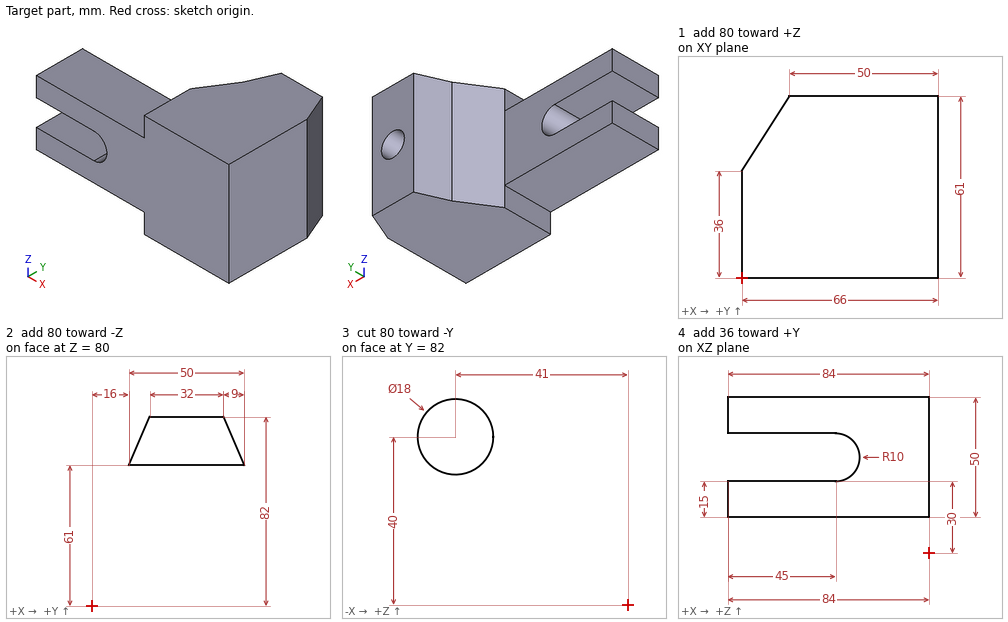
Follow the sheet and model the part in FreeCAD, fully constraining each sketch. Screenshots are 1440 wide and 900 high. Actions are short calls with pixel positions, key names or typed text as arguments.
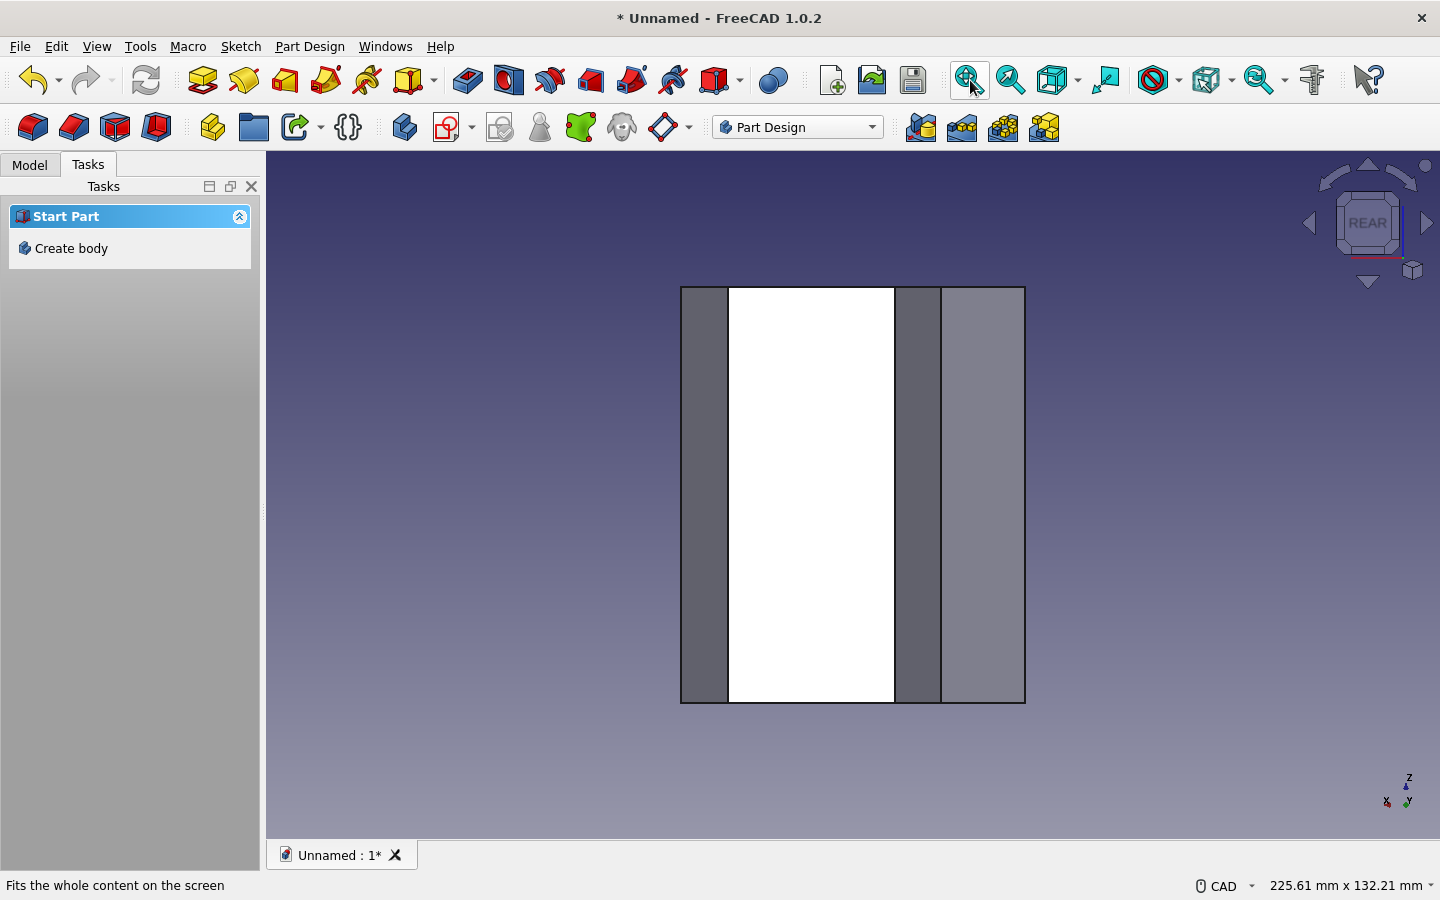
click(811, 375)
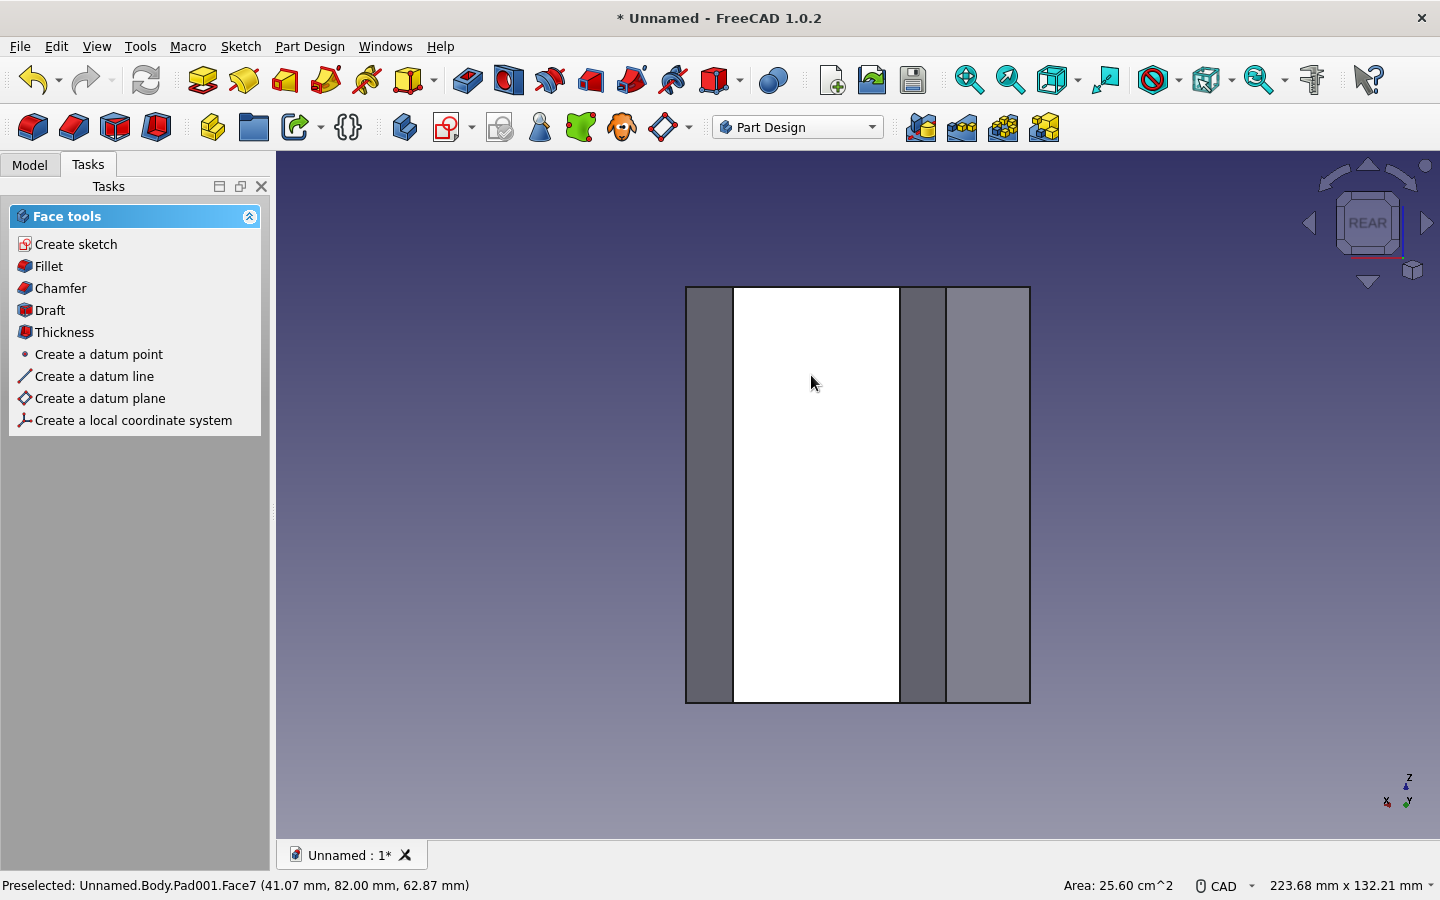
click(446, 128)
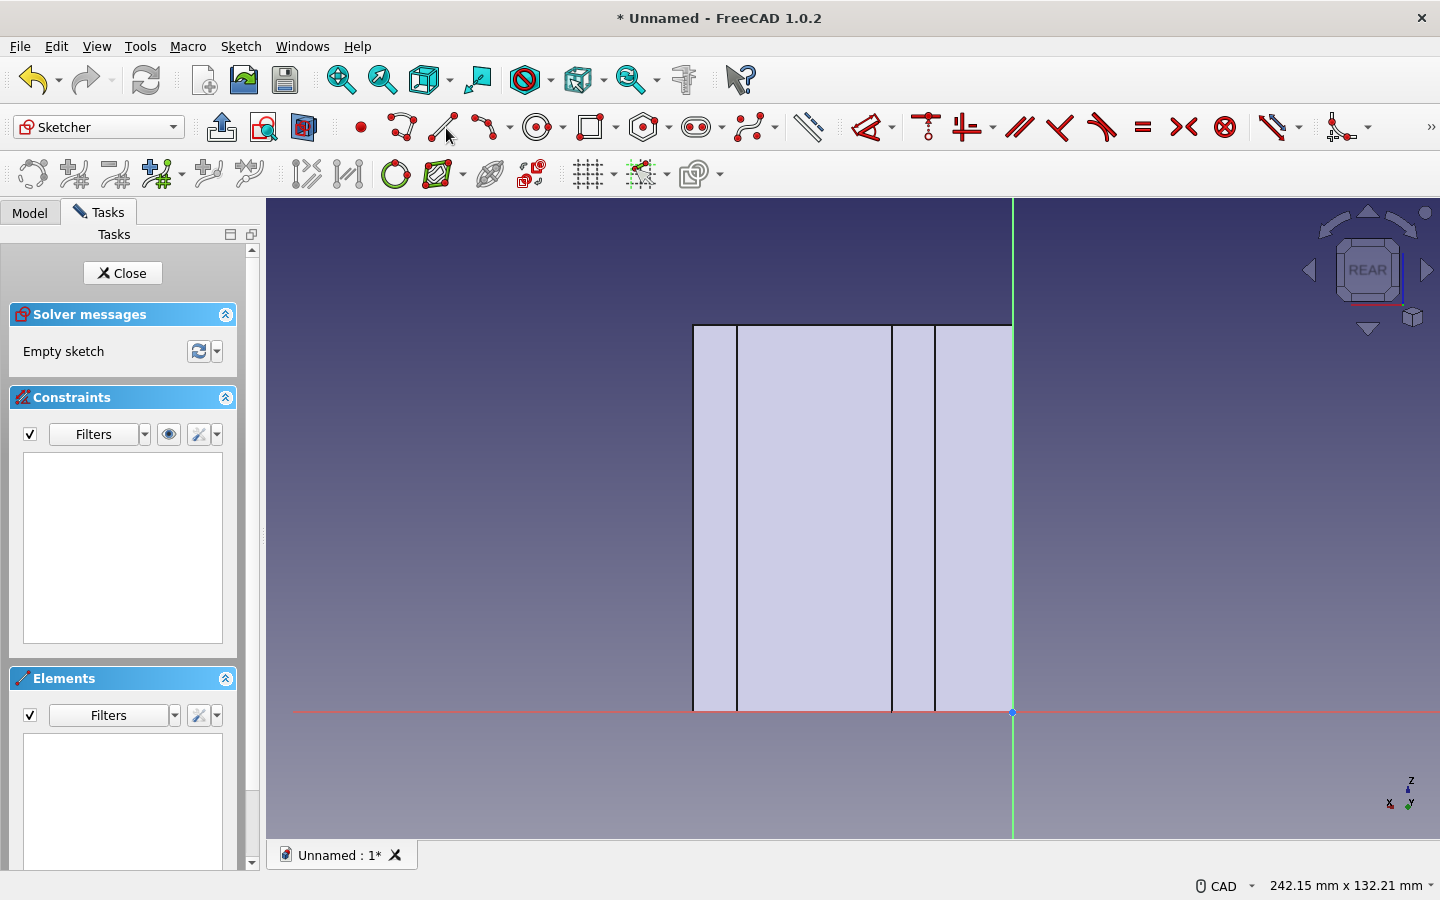
scroll(822, 518, up, 8)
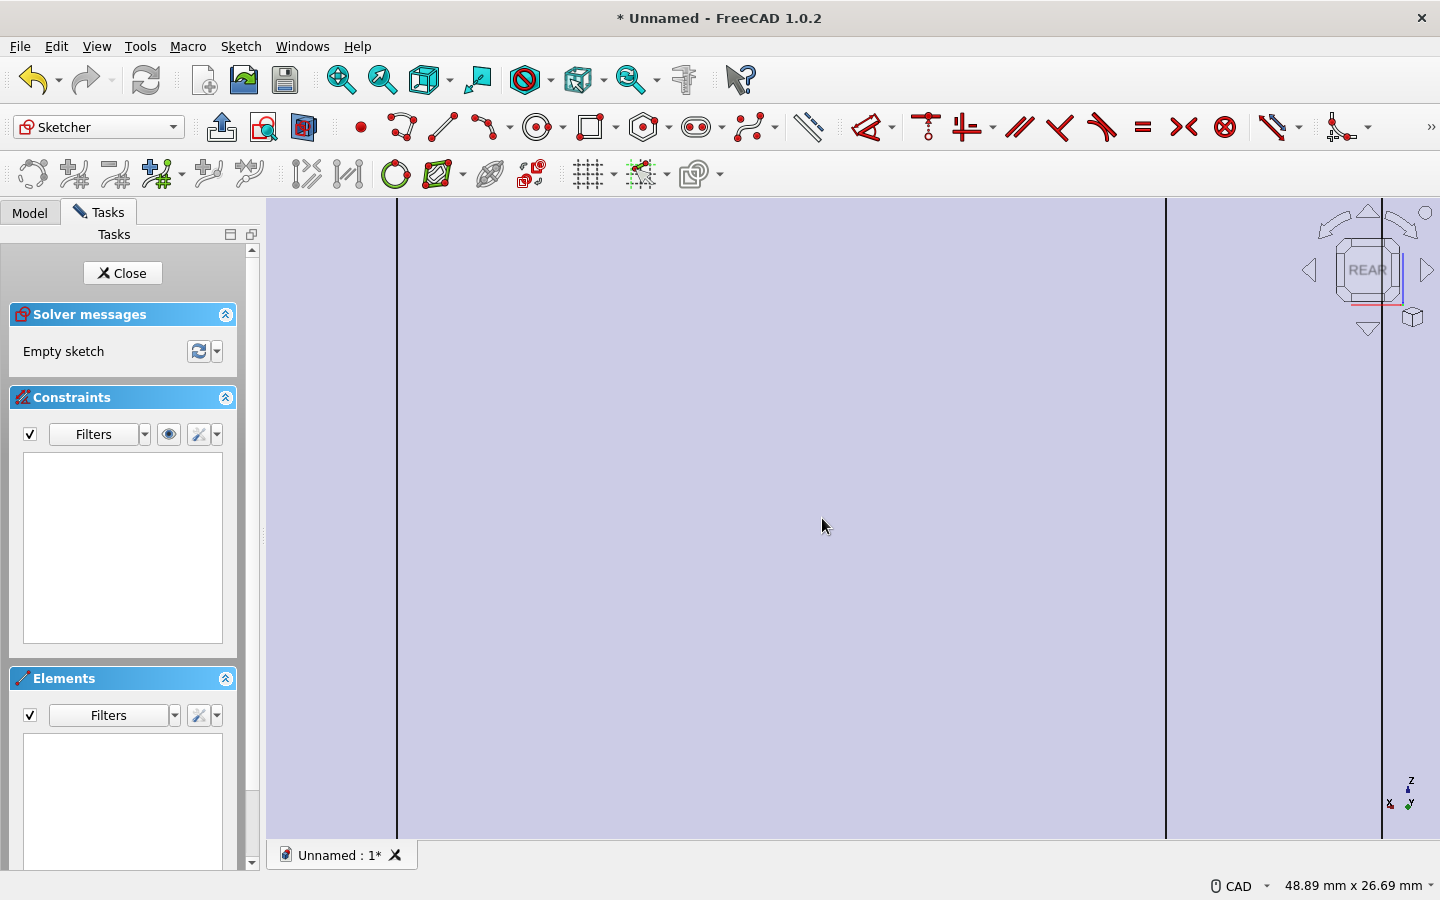
key(g)
key(c)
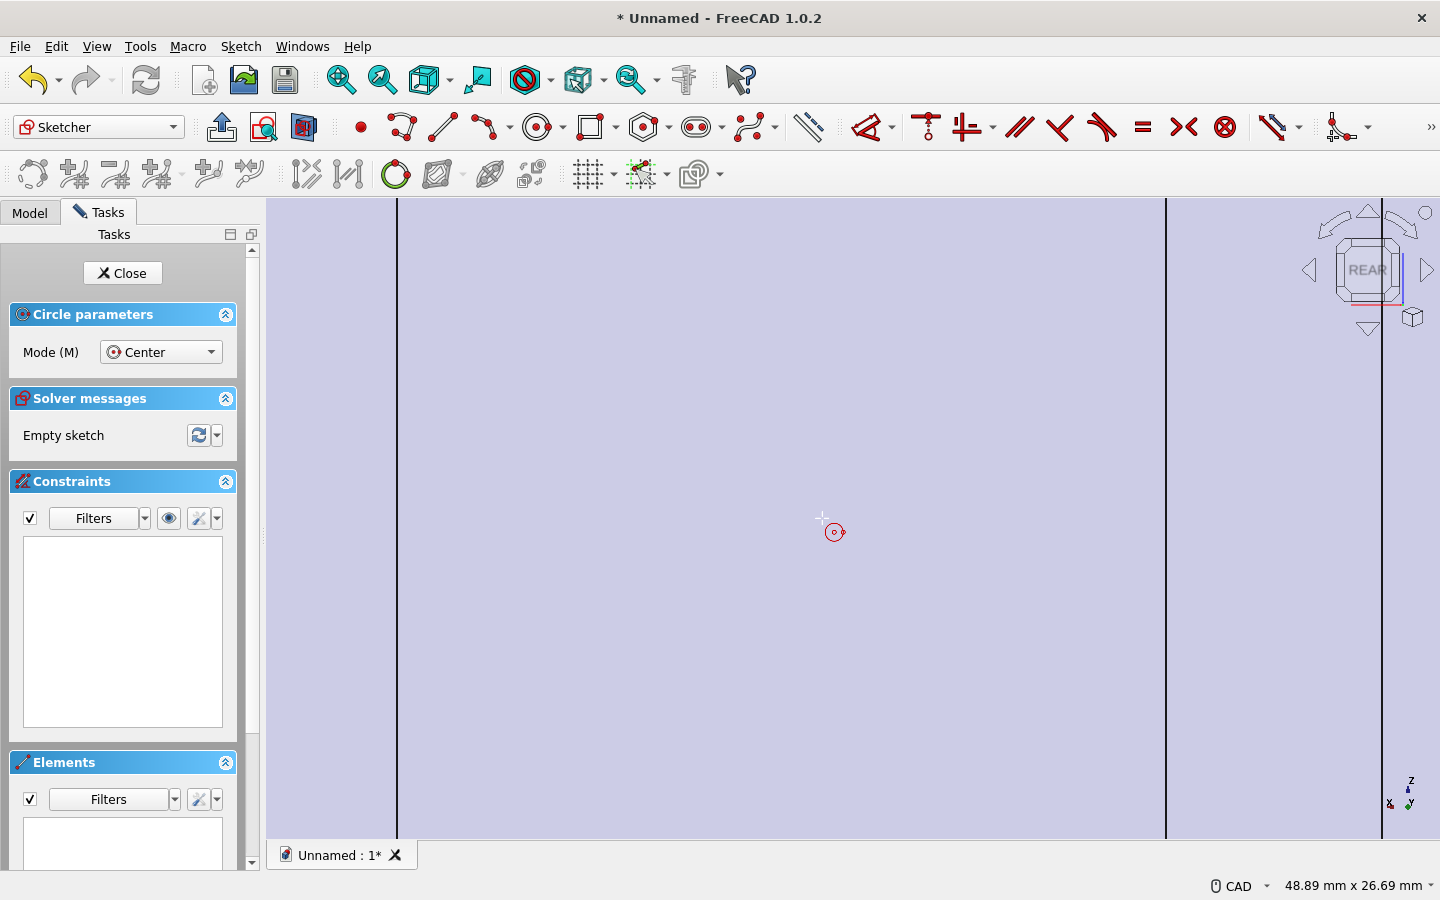
click(782, 518)
move(934, 366)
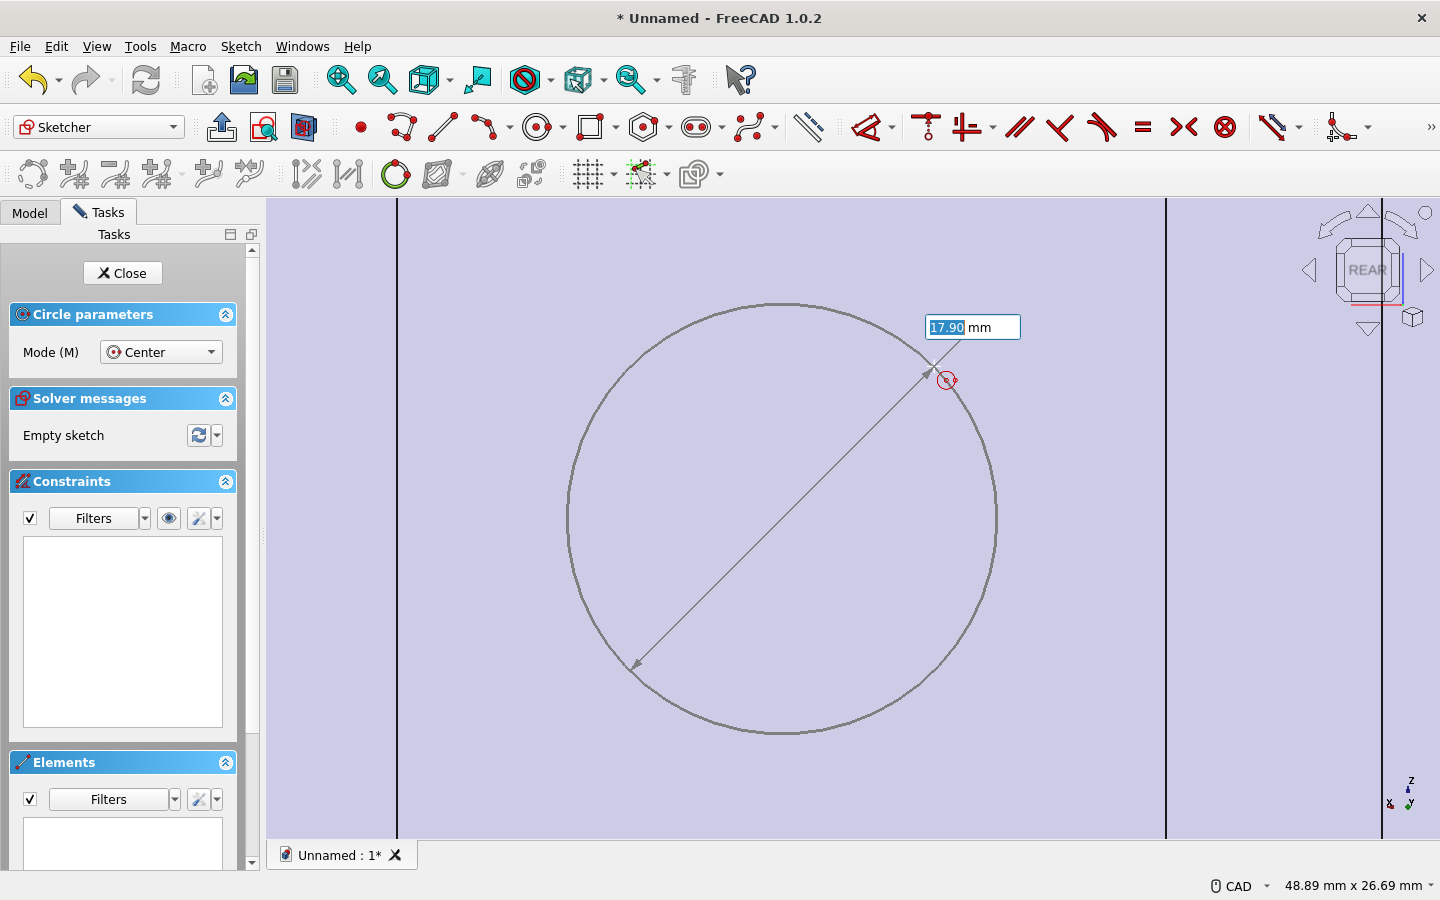
text(18)
key(Return)
key(Escape)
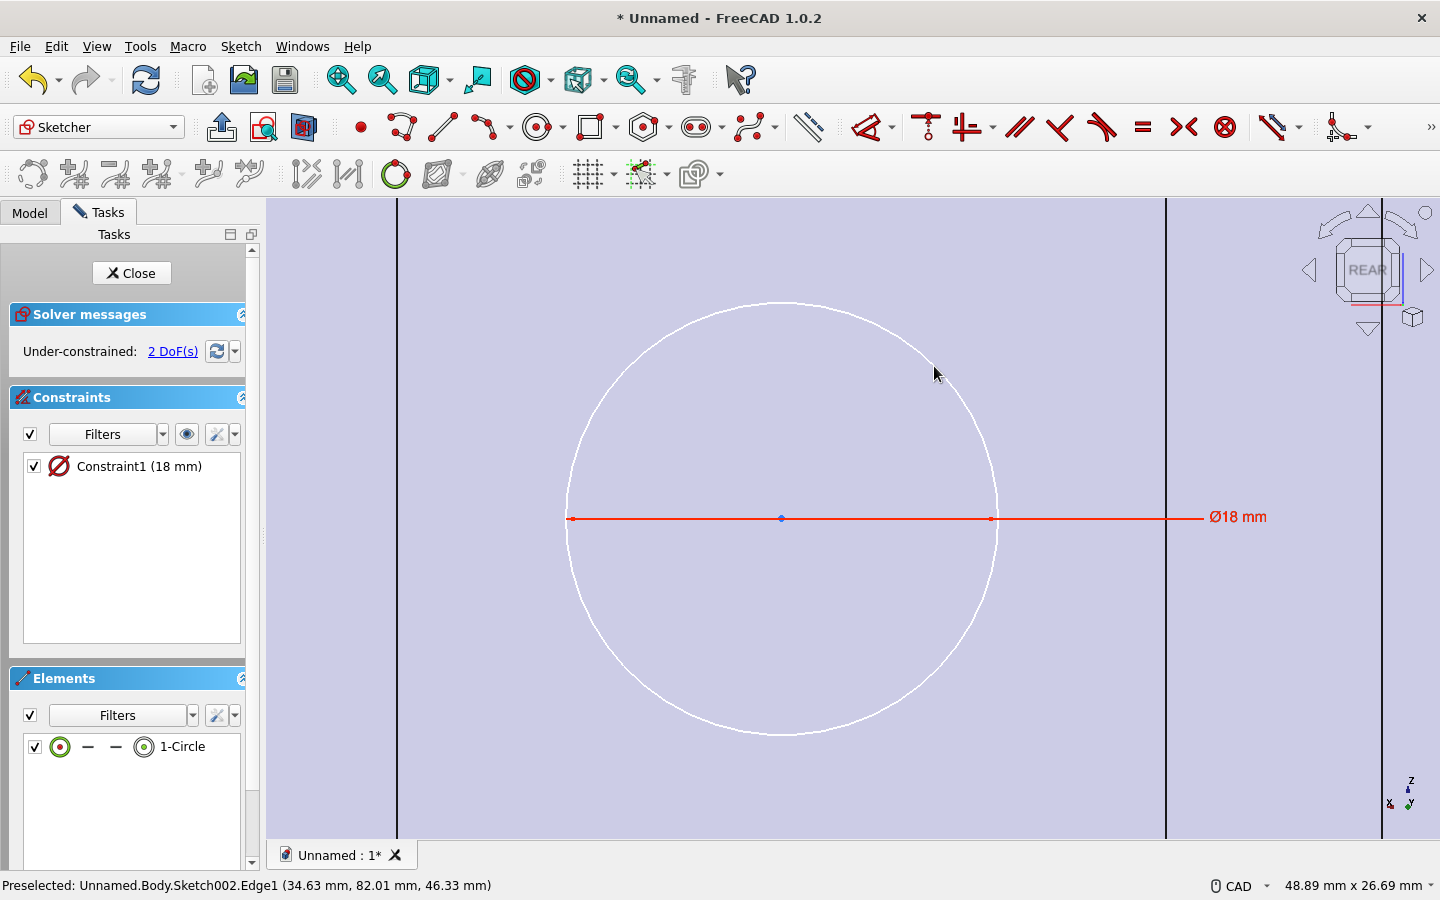
key(d)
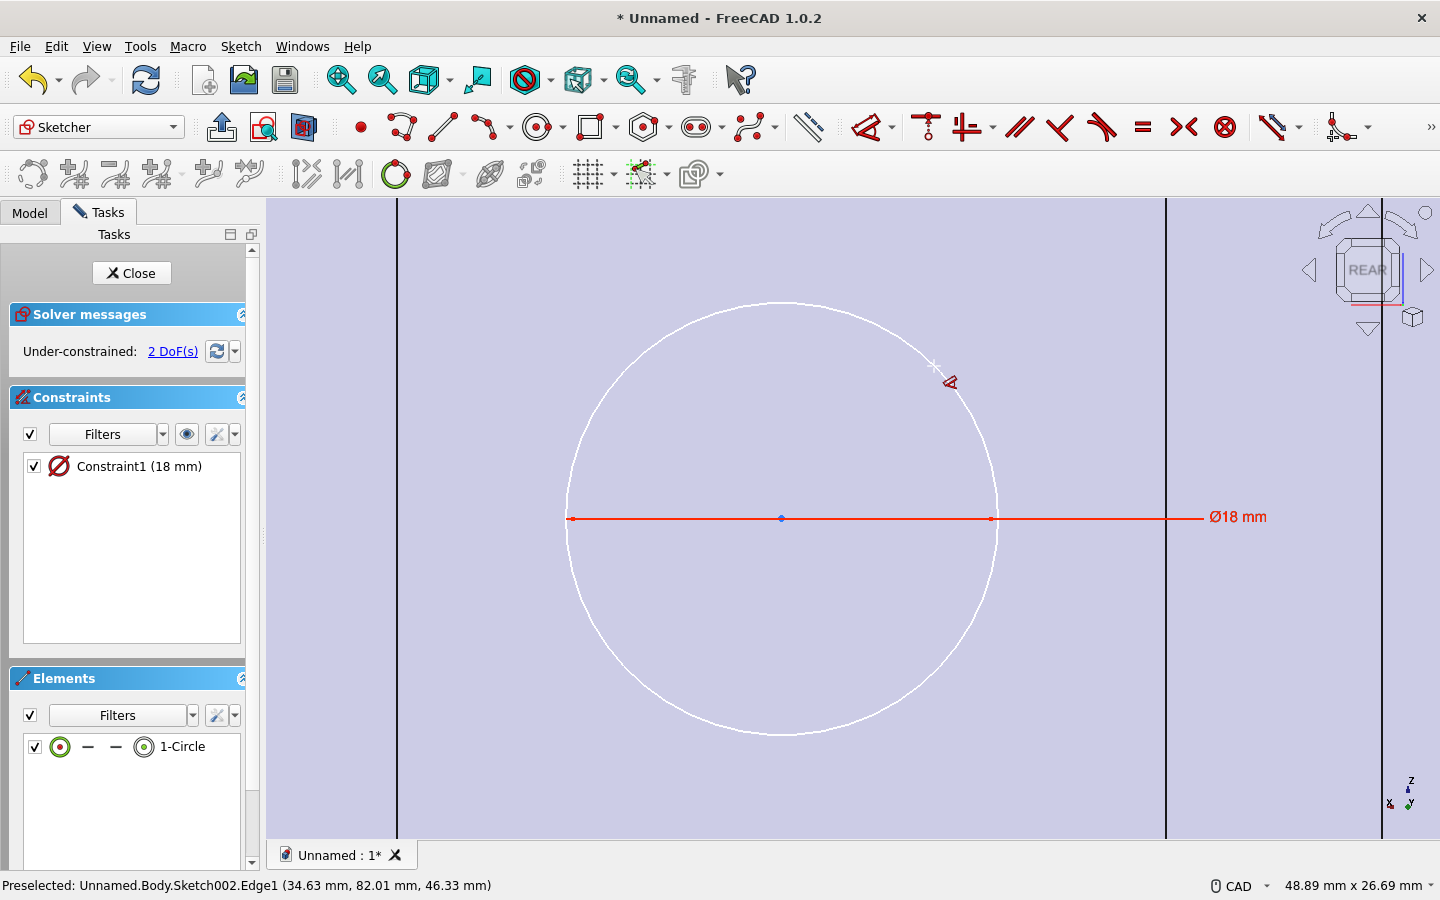
click(782, 519)
click(1029, 485)